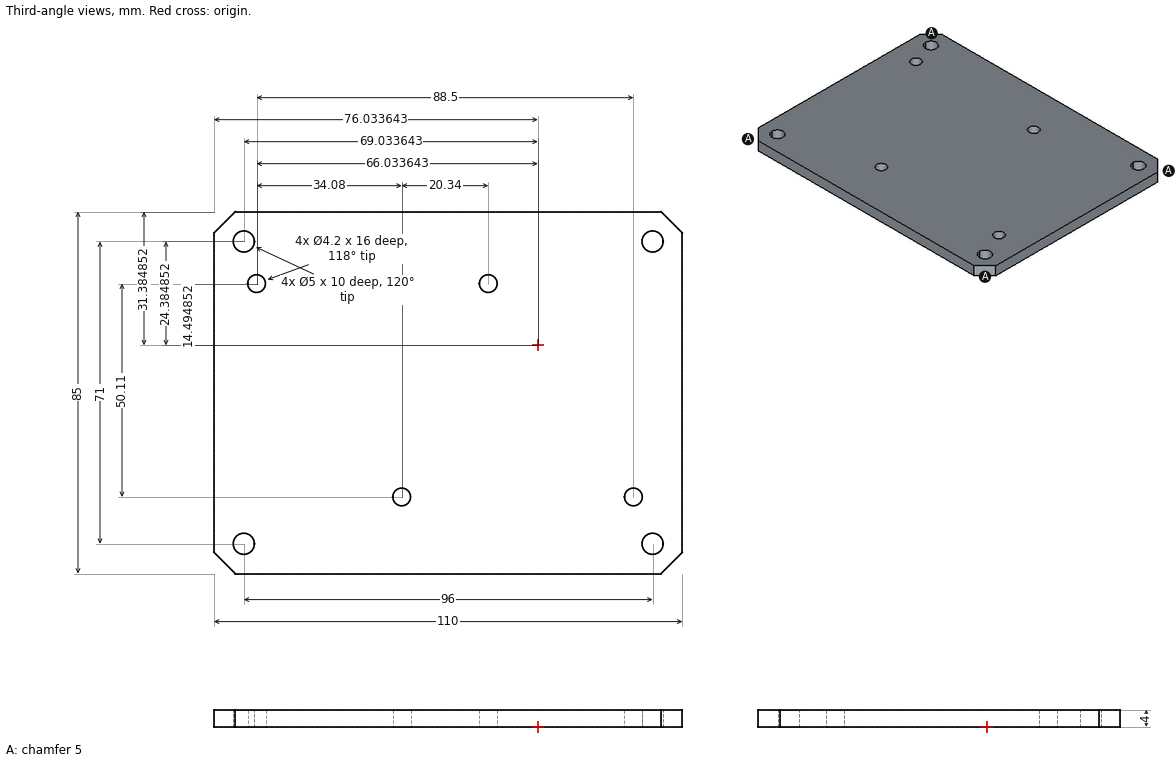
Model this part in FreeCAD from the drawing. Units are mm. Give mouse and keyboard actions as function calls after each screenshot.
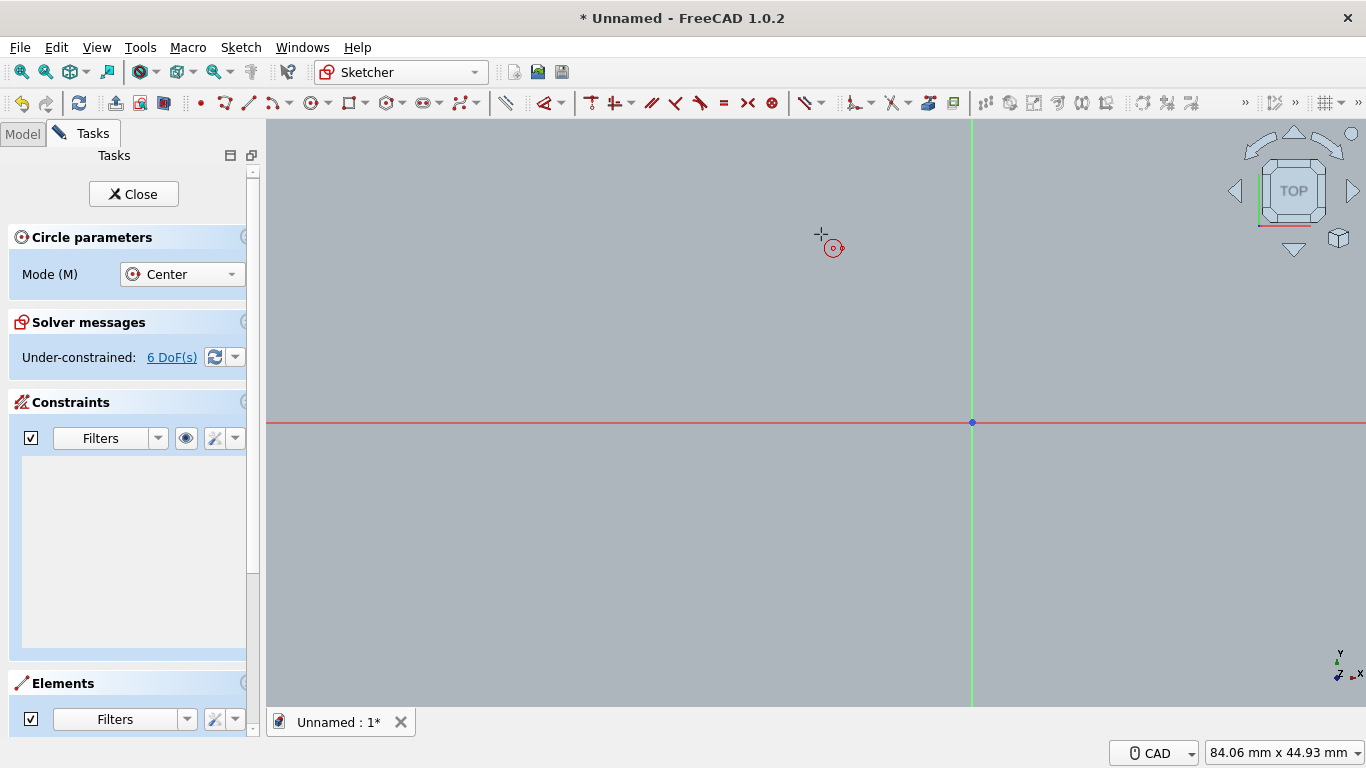
click(820, 233)
click(840, 214)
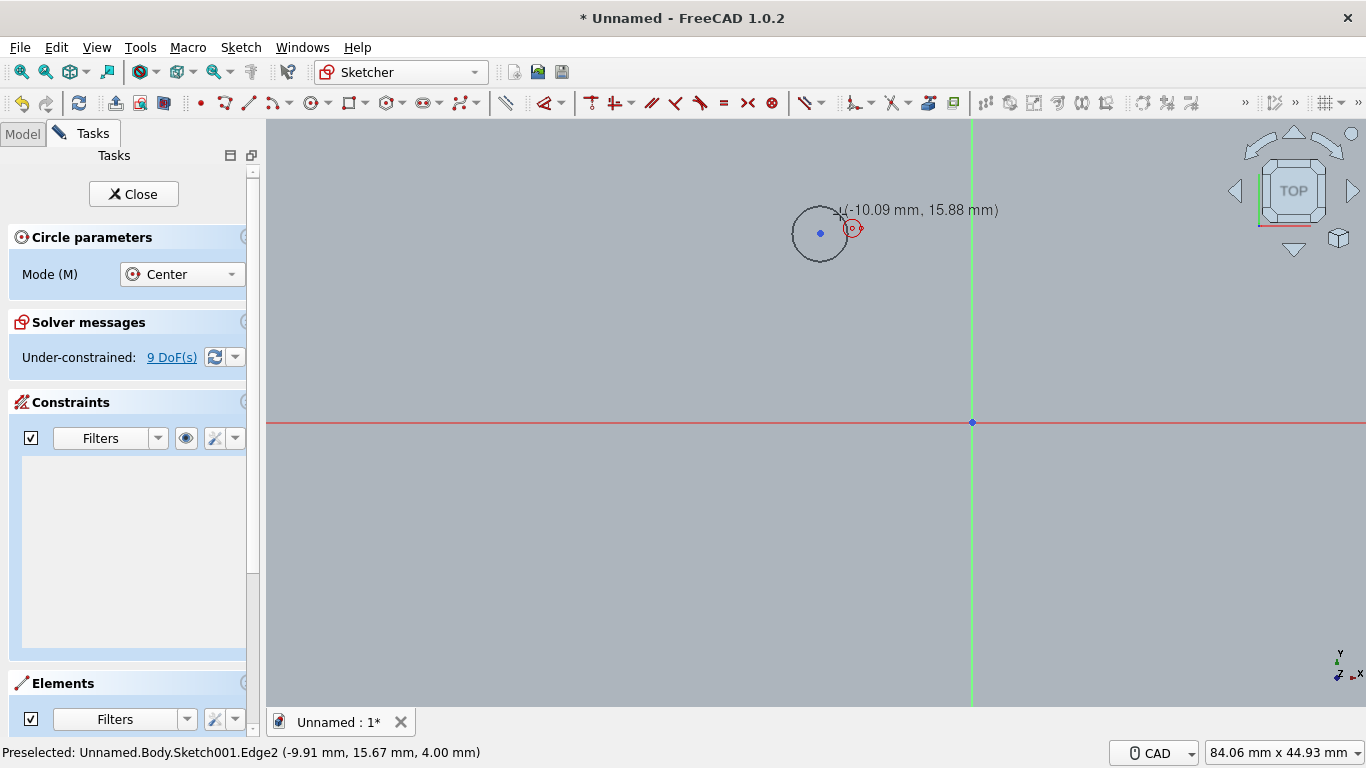
scroll(821, 233, down, 3)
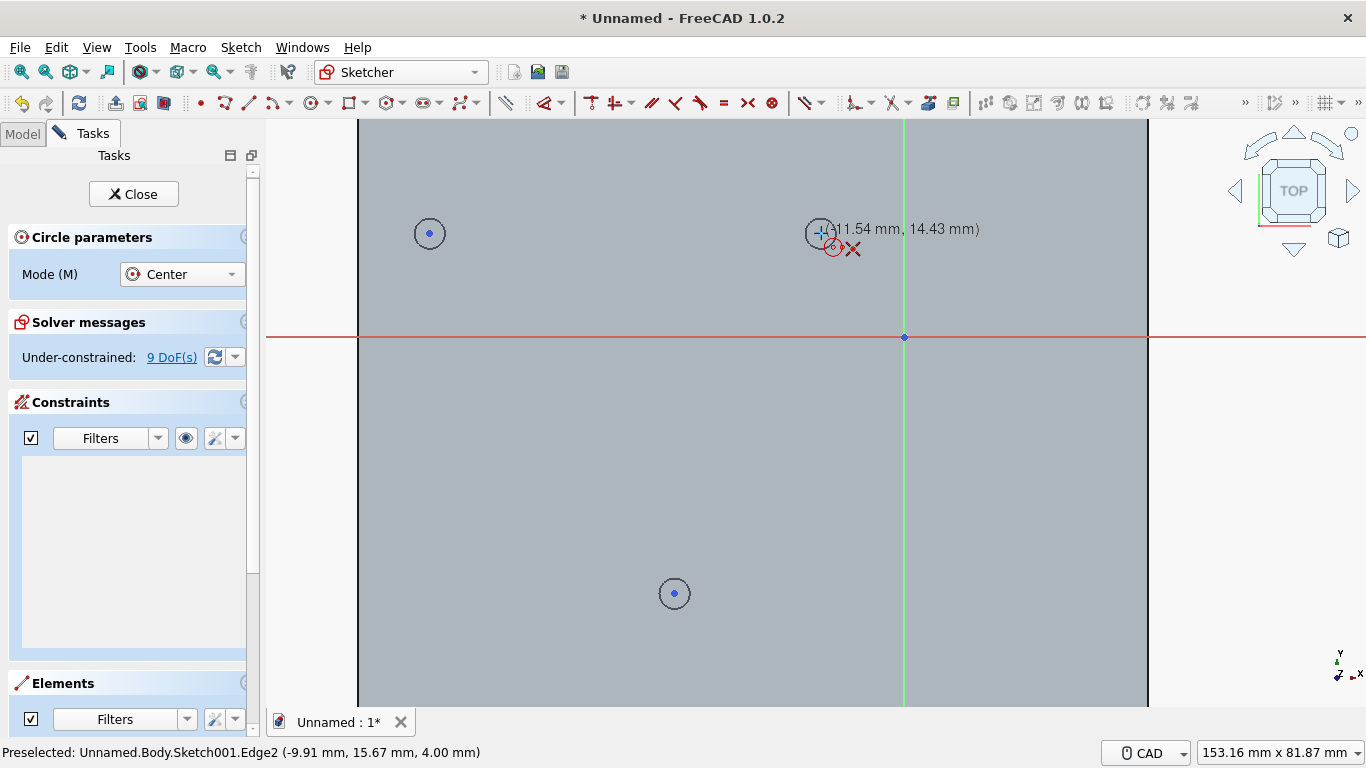
scroll(1065, 593, up, 3)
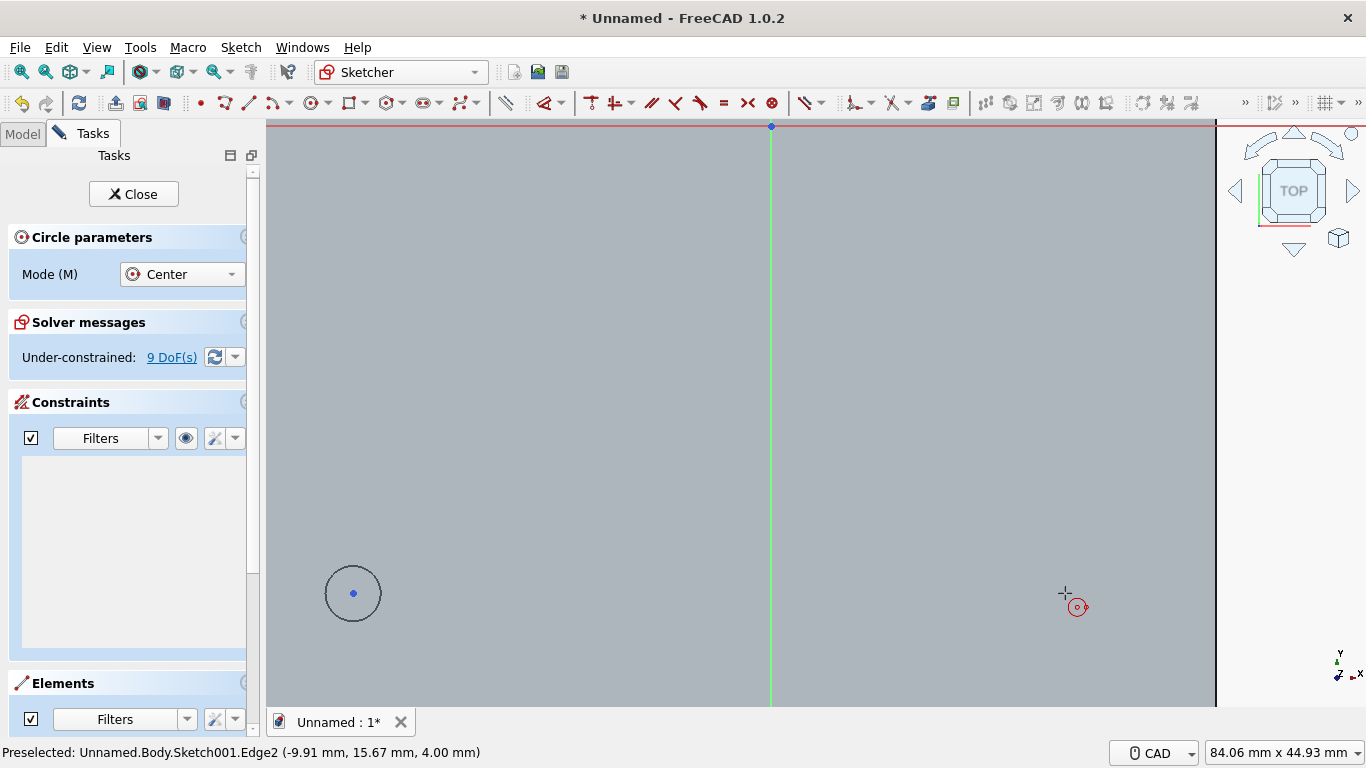
click(1065, 592)
click(1085, 573)
key(Escape)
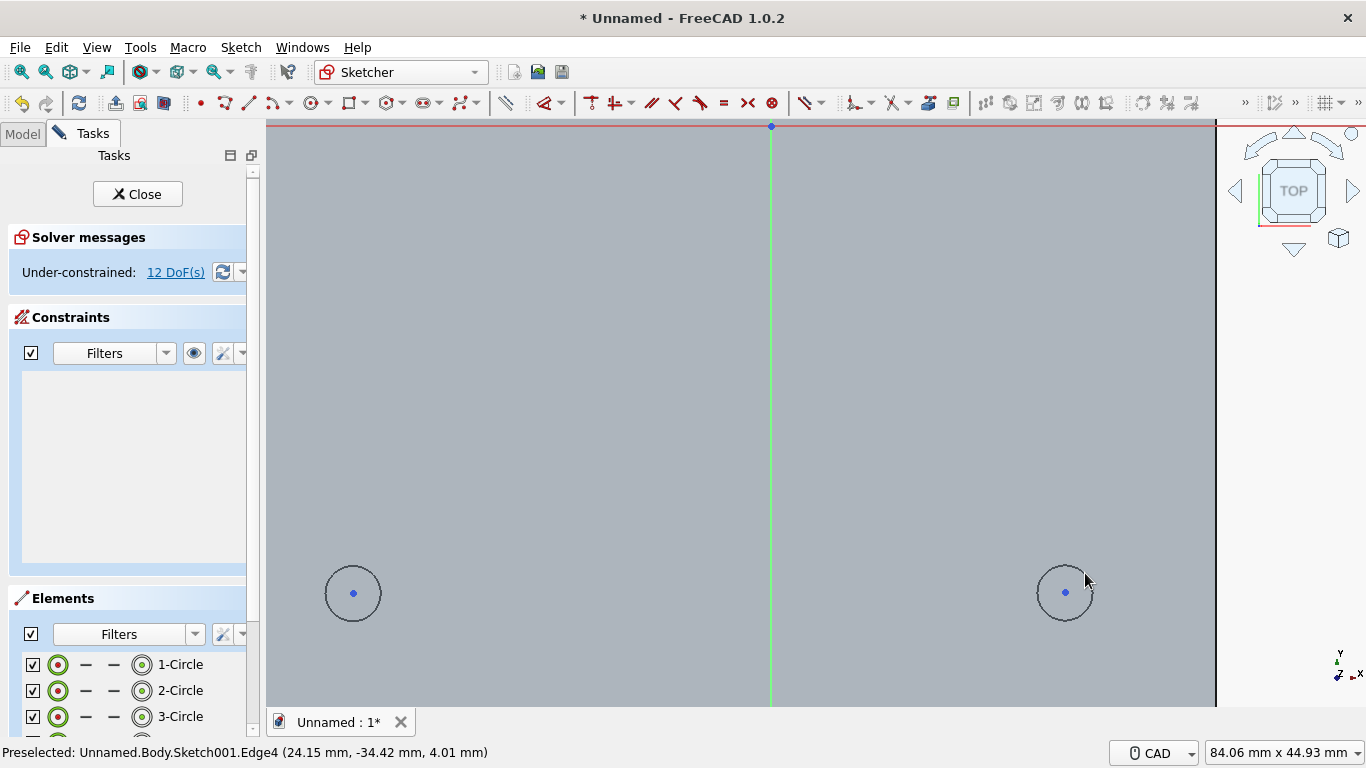
scroll(1065, 594, down, 3)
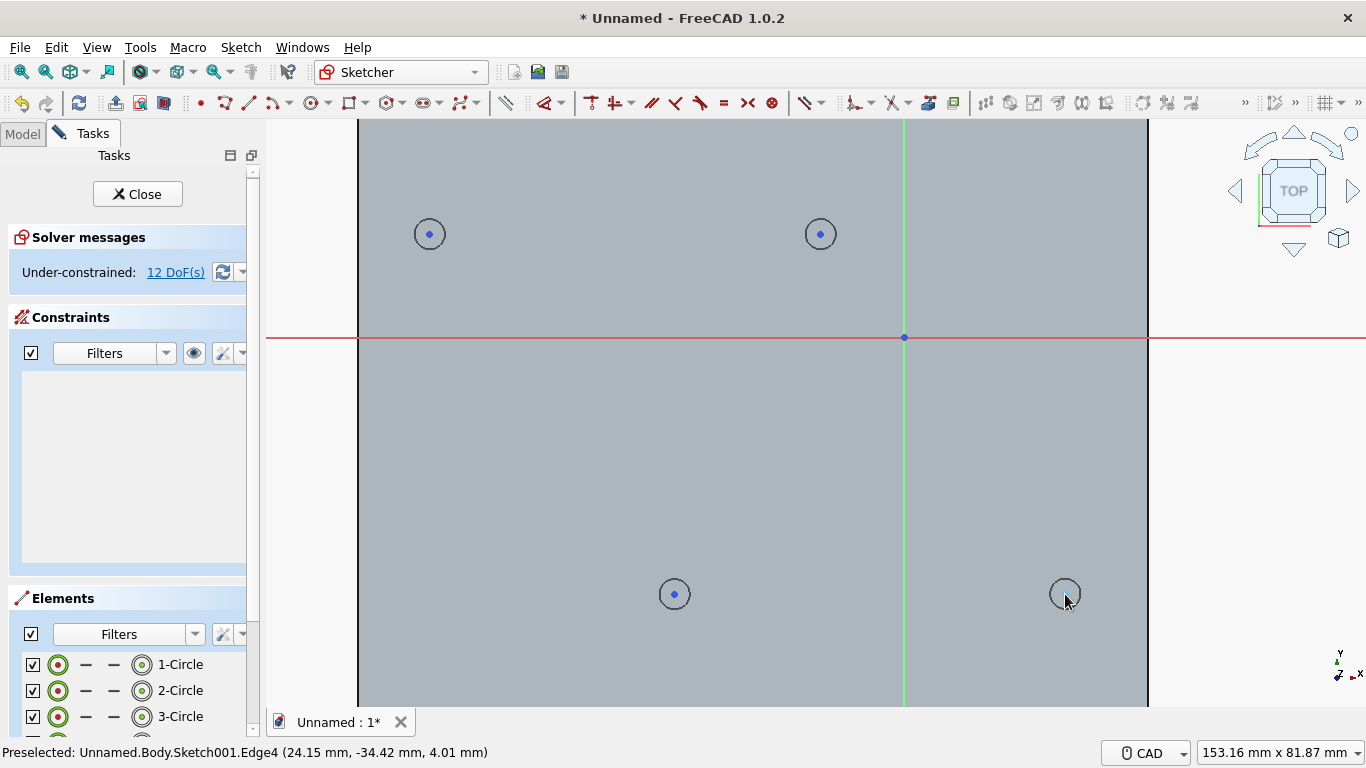
click(440, 223)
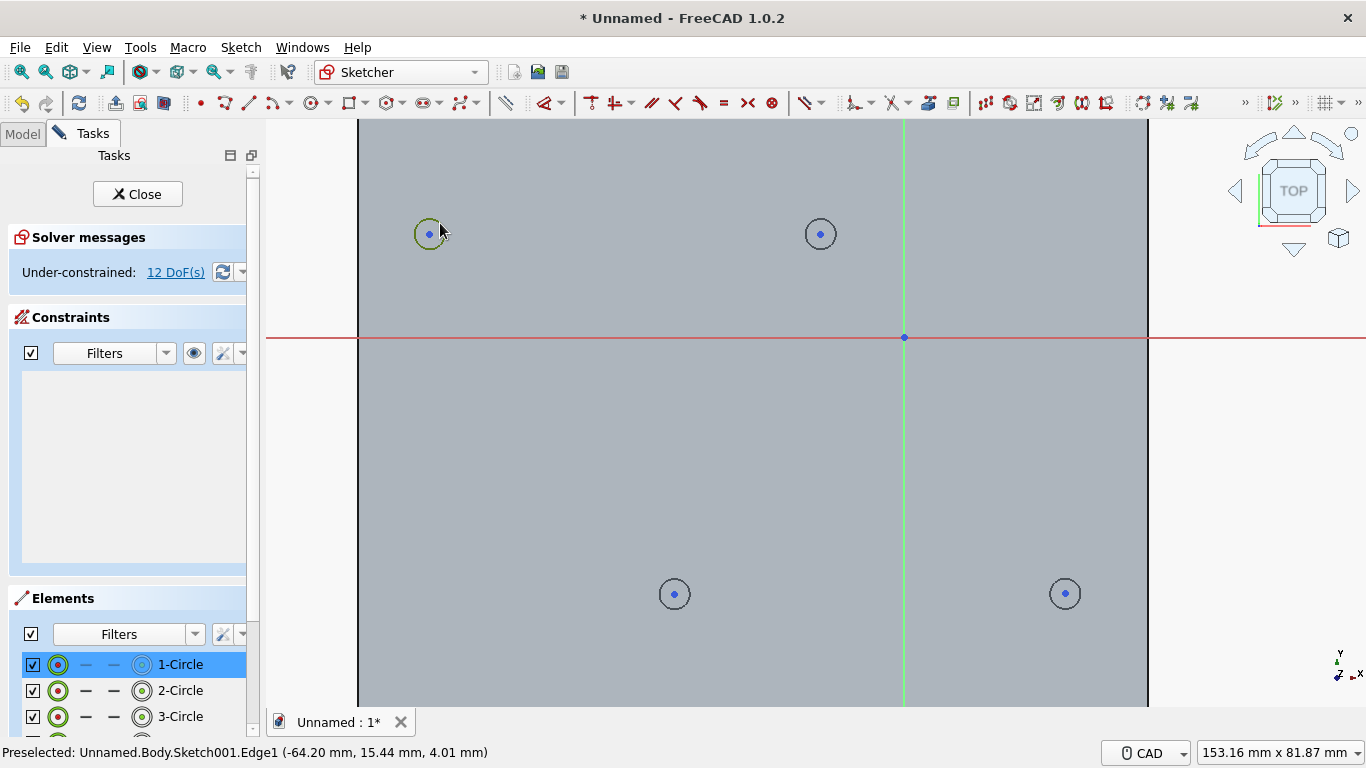
click(685, 583)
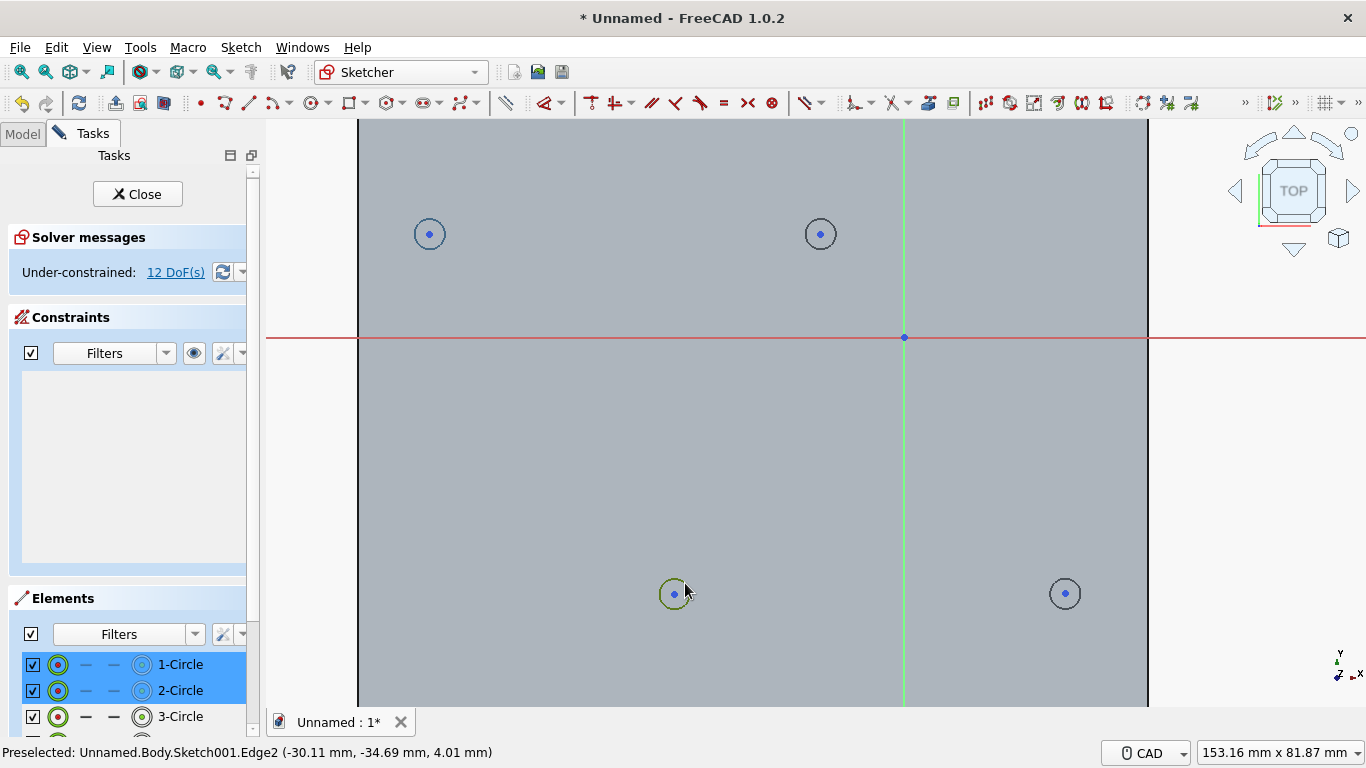
click(831, 223)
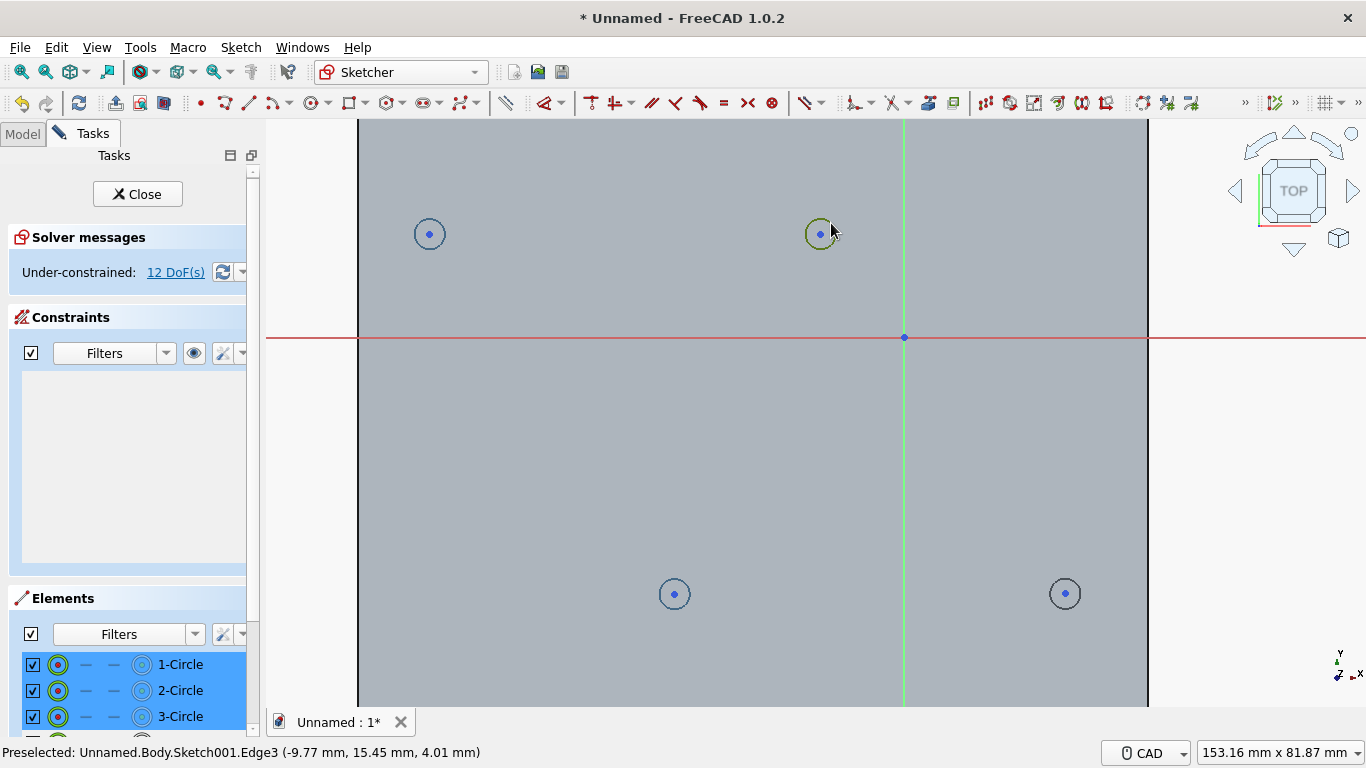
click(1076, 583)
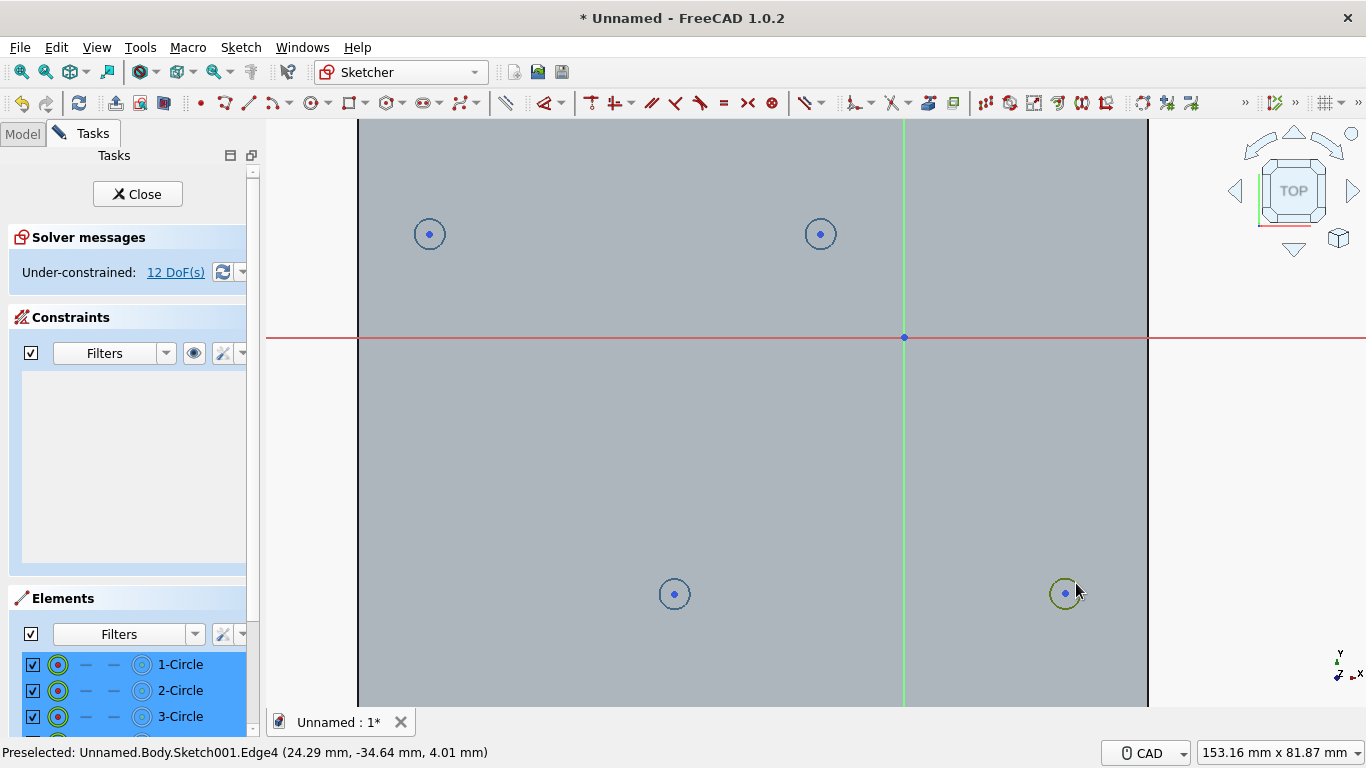
click(724, 104)